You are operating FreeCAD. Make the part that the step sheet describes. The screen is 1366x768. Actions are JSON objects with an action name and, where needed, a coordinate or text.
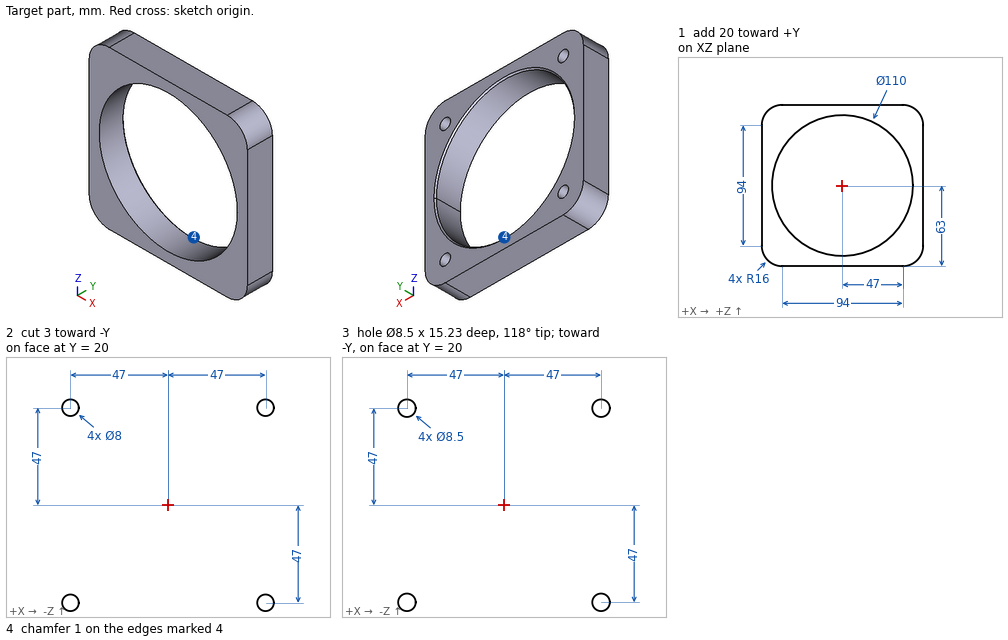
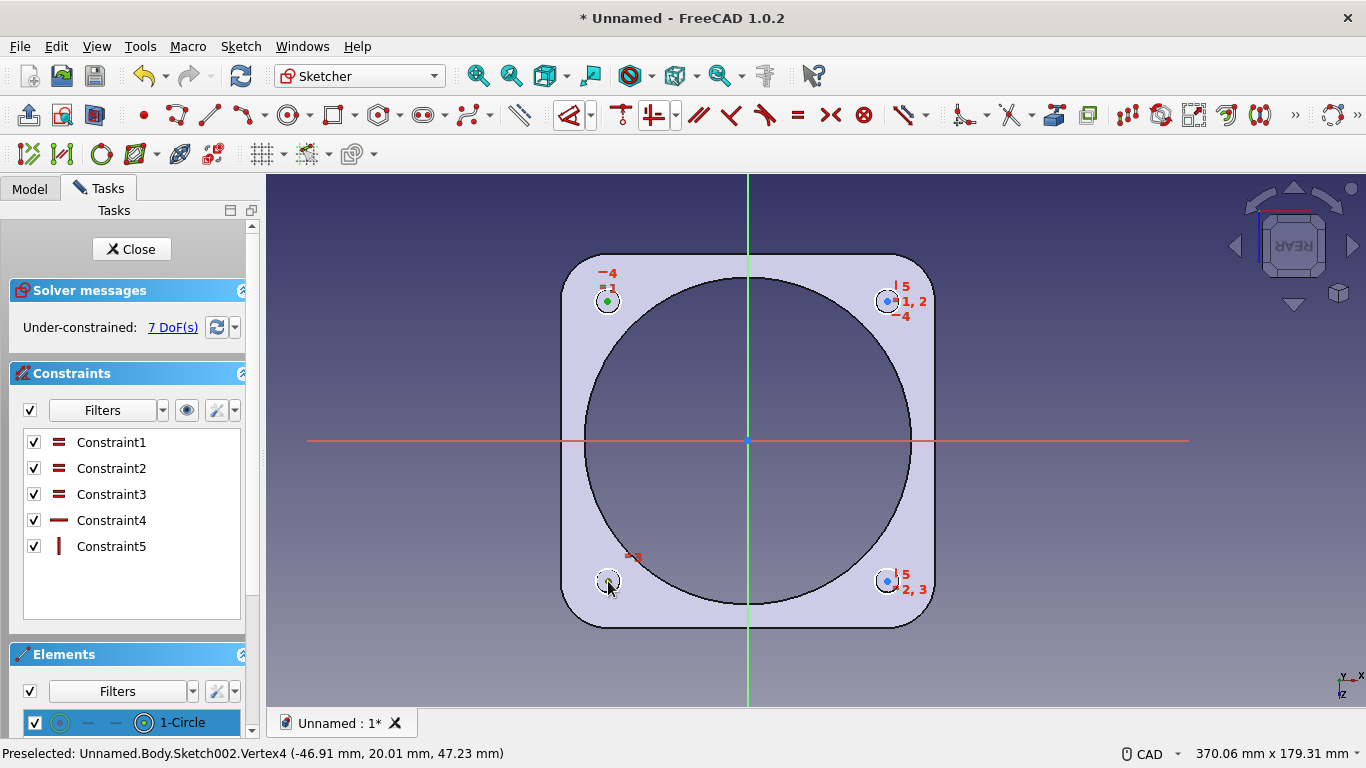
{"action": "key", "text": "v"}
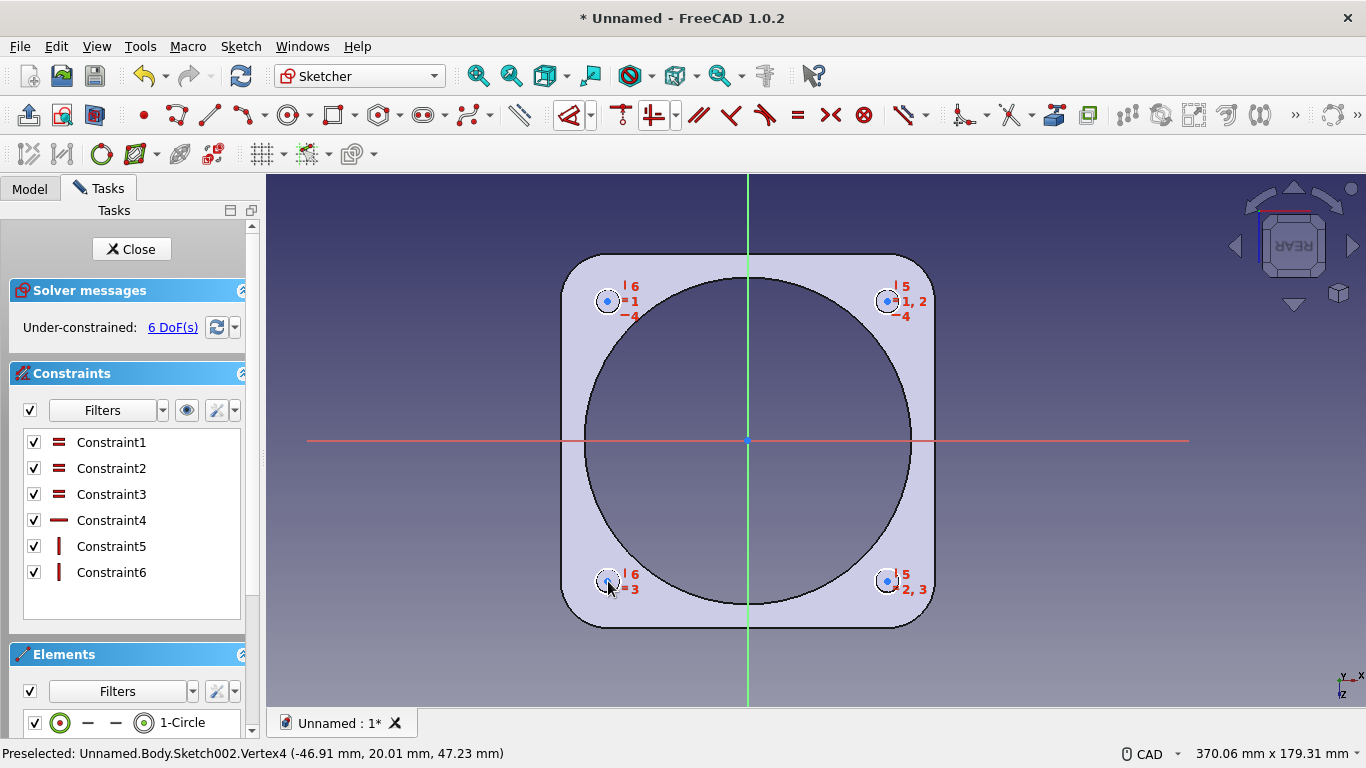
{"action": "left_click", "coordinate": [887, 581]}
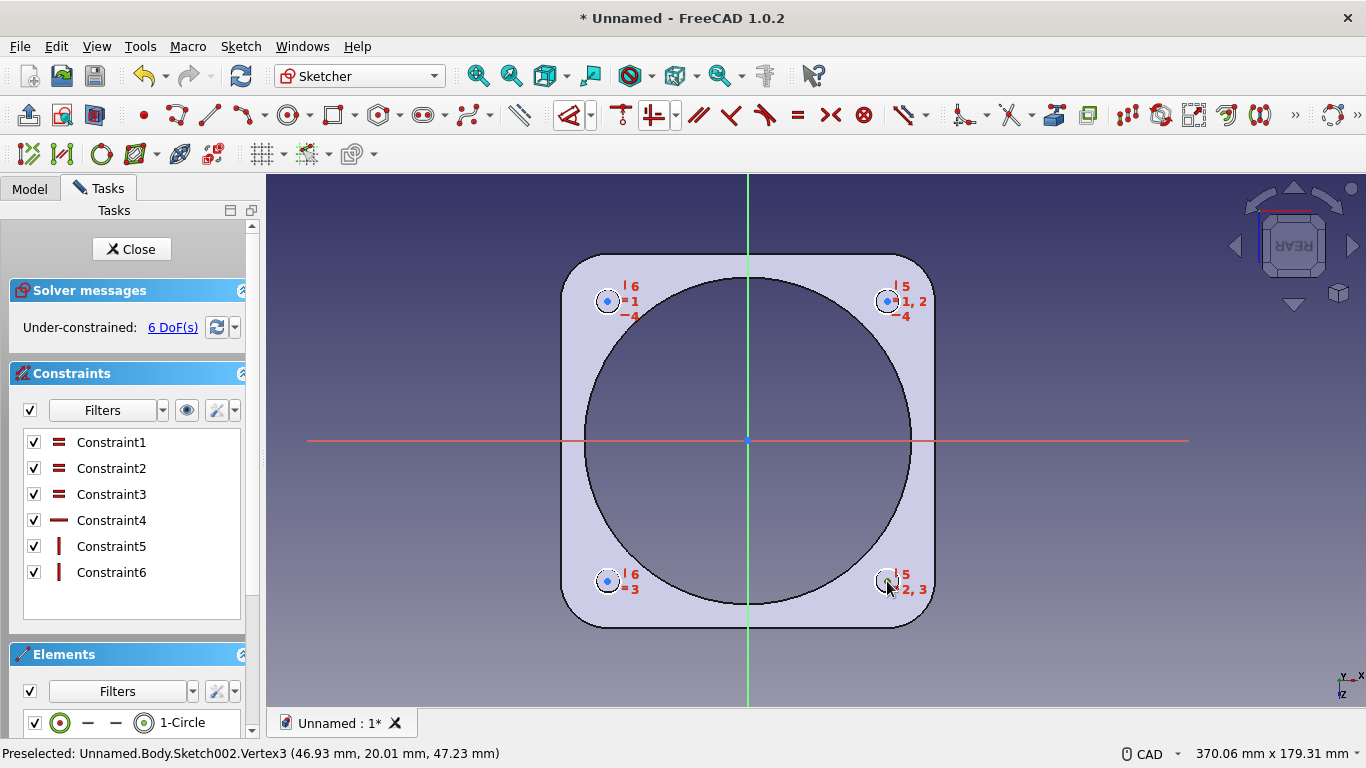
{"action": "left_click", "coordinate": [608, 581]}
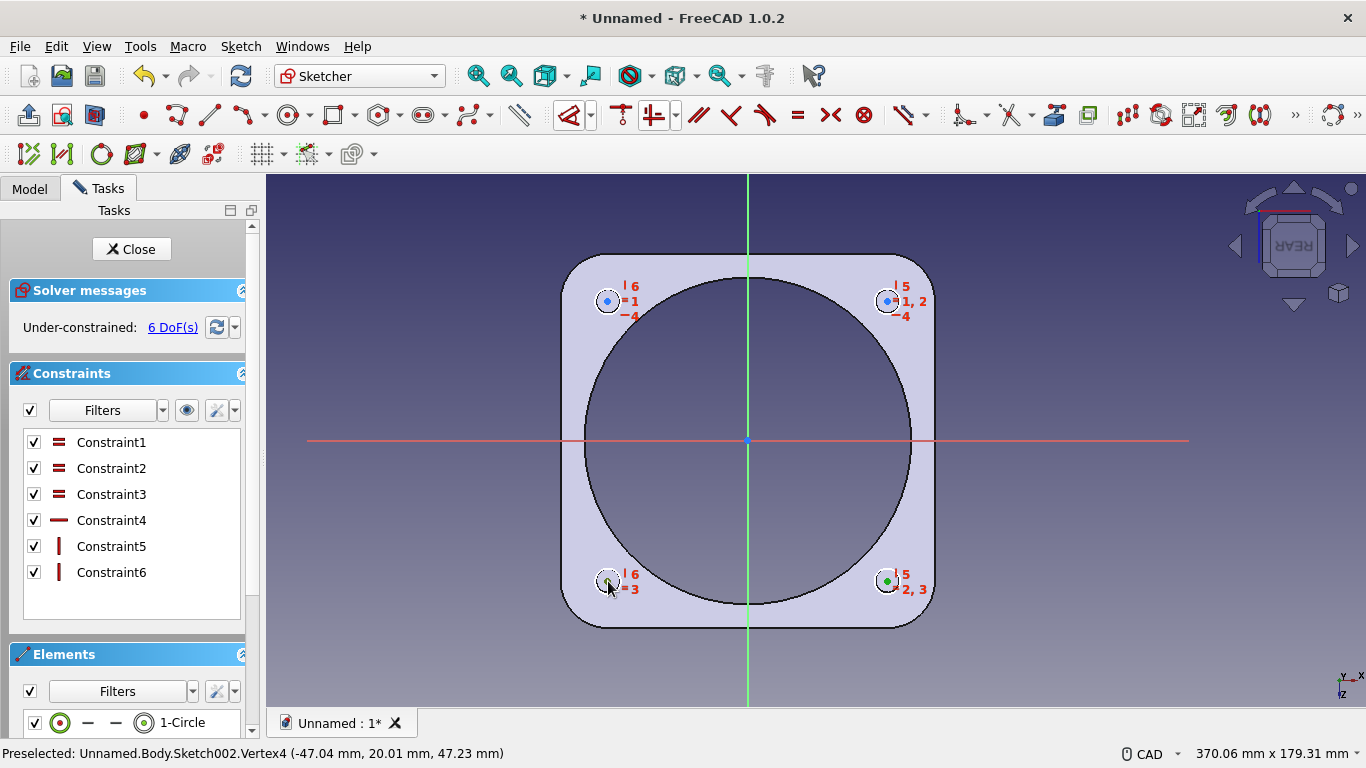
{"action": "key", "text": "h"}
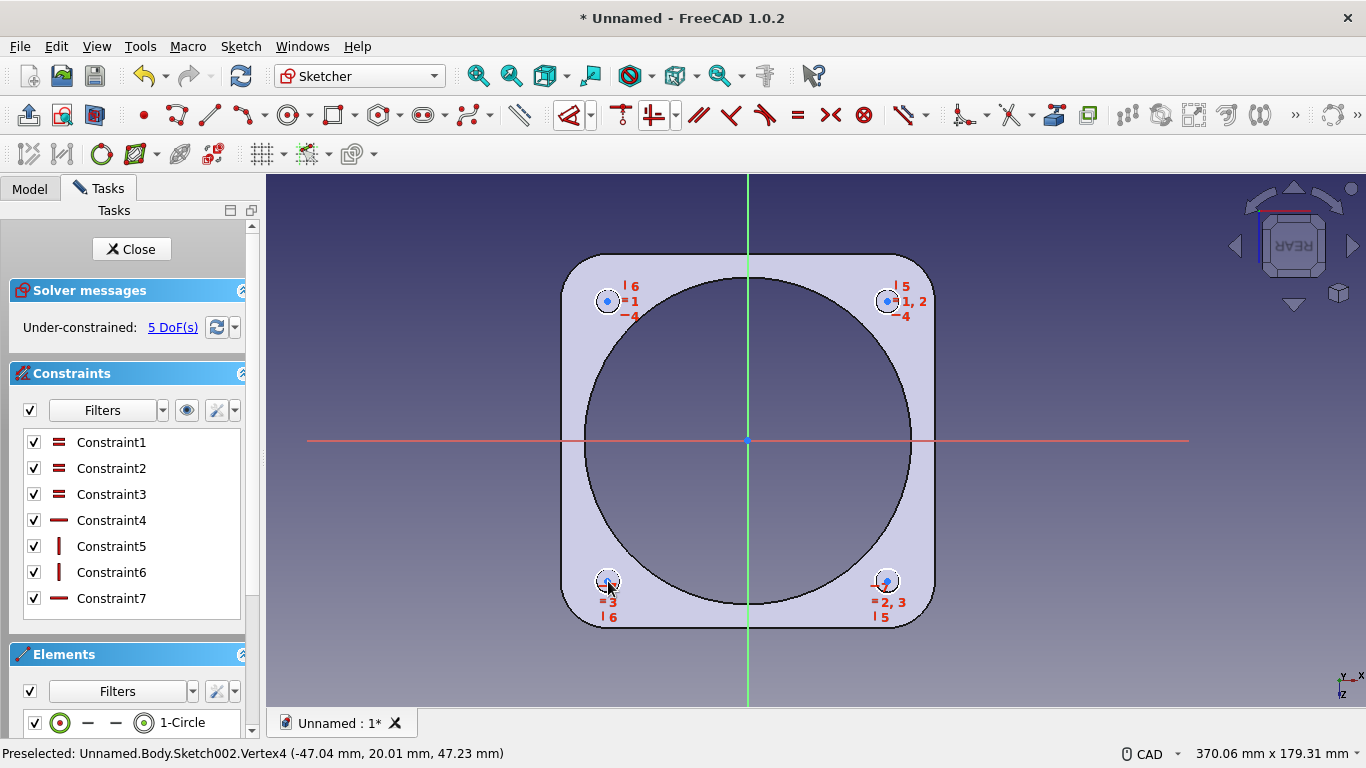
{"action": "scroll", "coordinate": [617, 292], "scroll_direction": "up", "scroll_amount": 3}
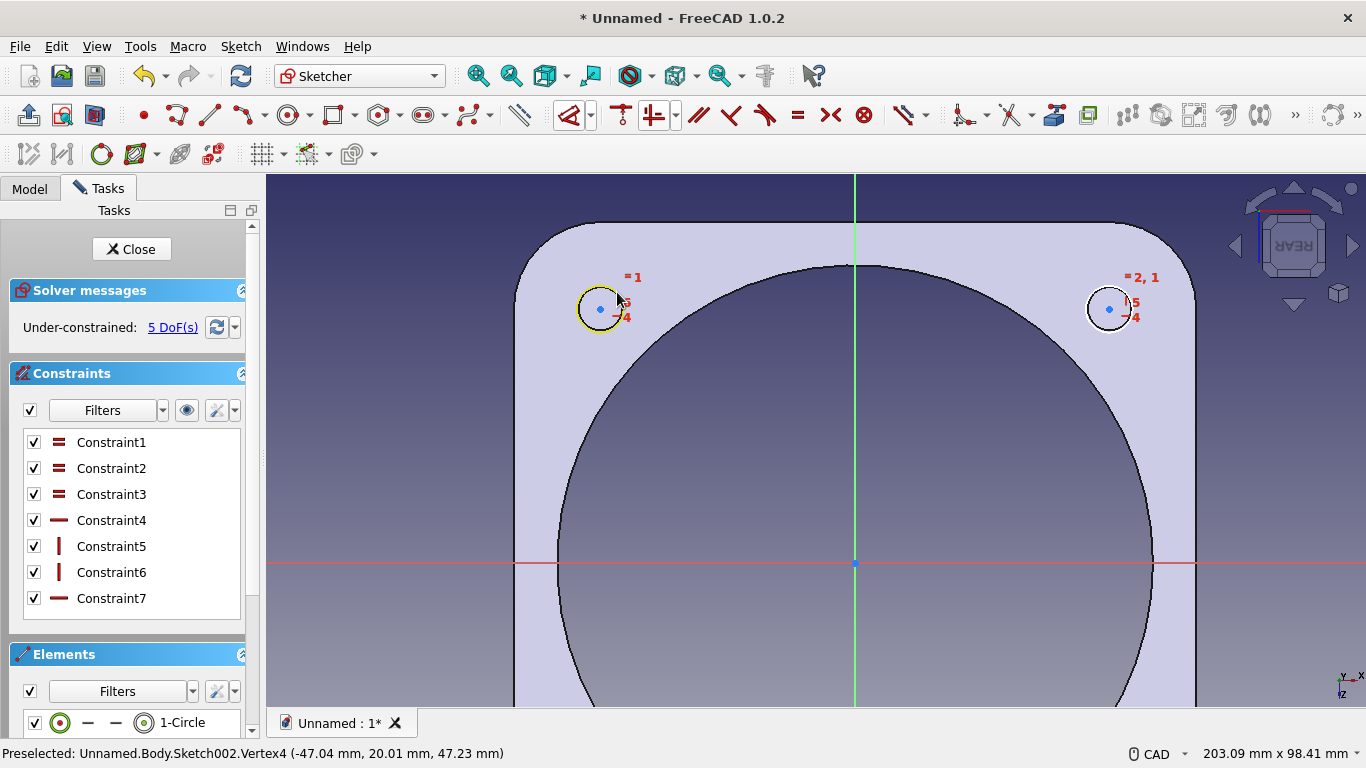
{"action": "left_click", "coordinate": [617, 293]}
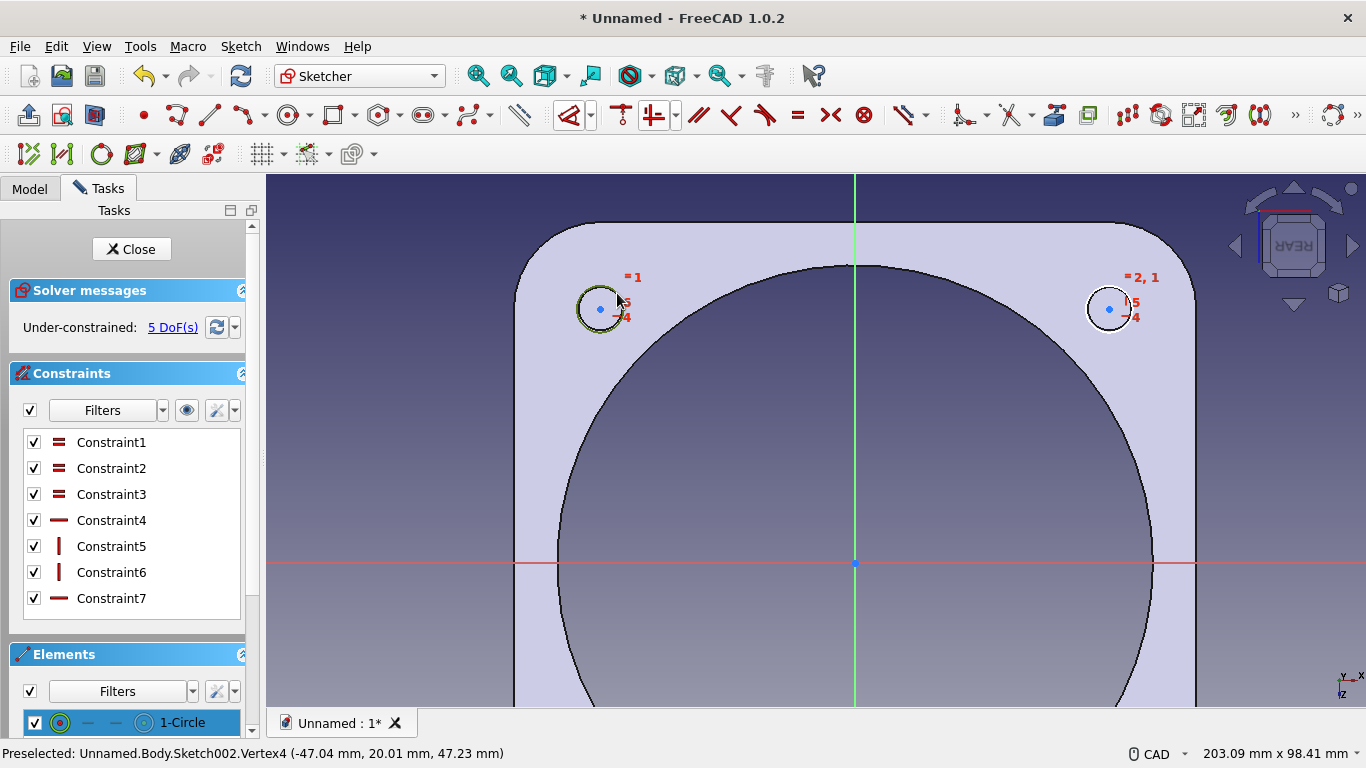
{"action": "key", "text": "k o"}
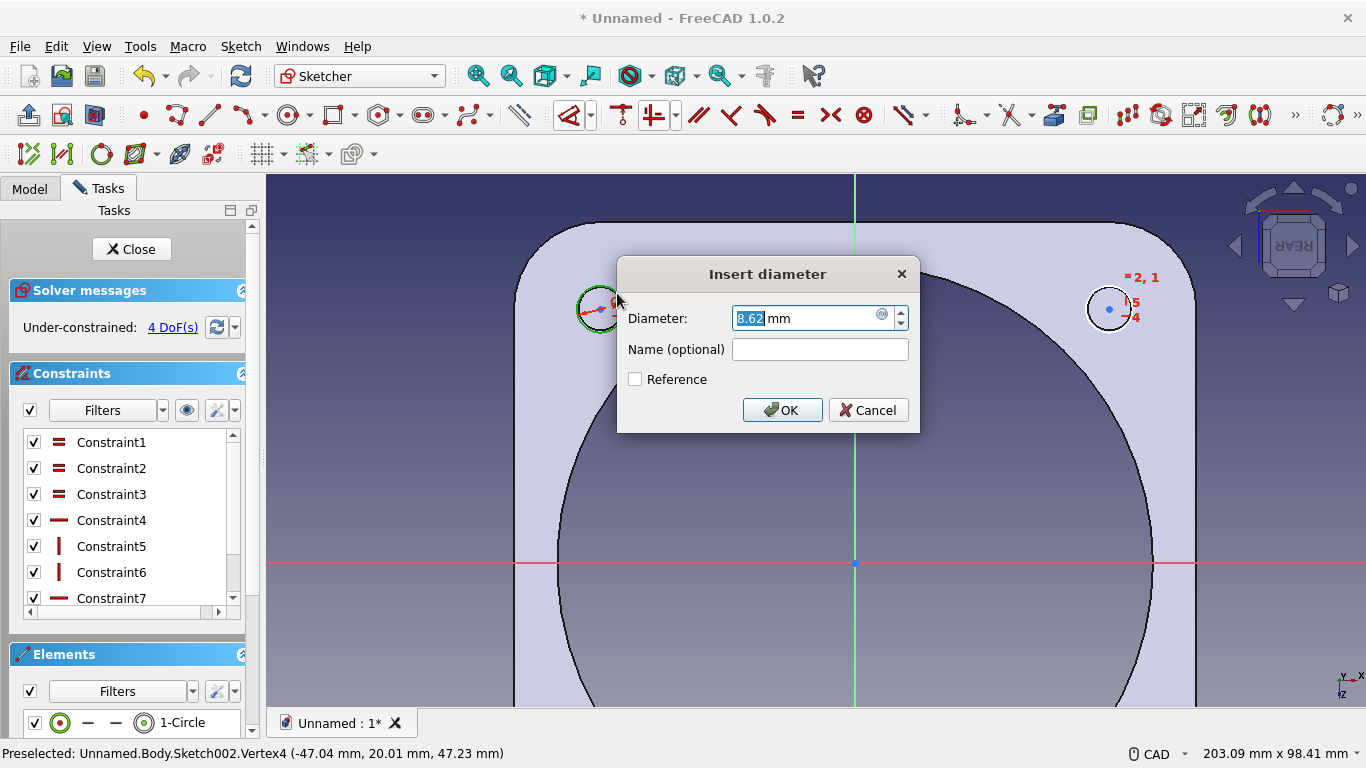
{"action": "type", "text": "8.5"}
{"action": "key", "text": "Return"}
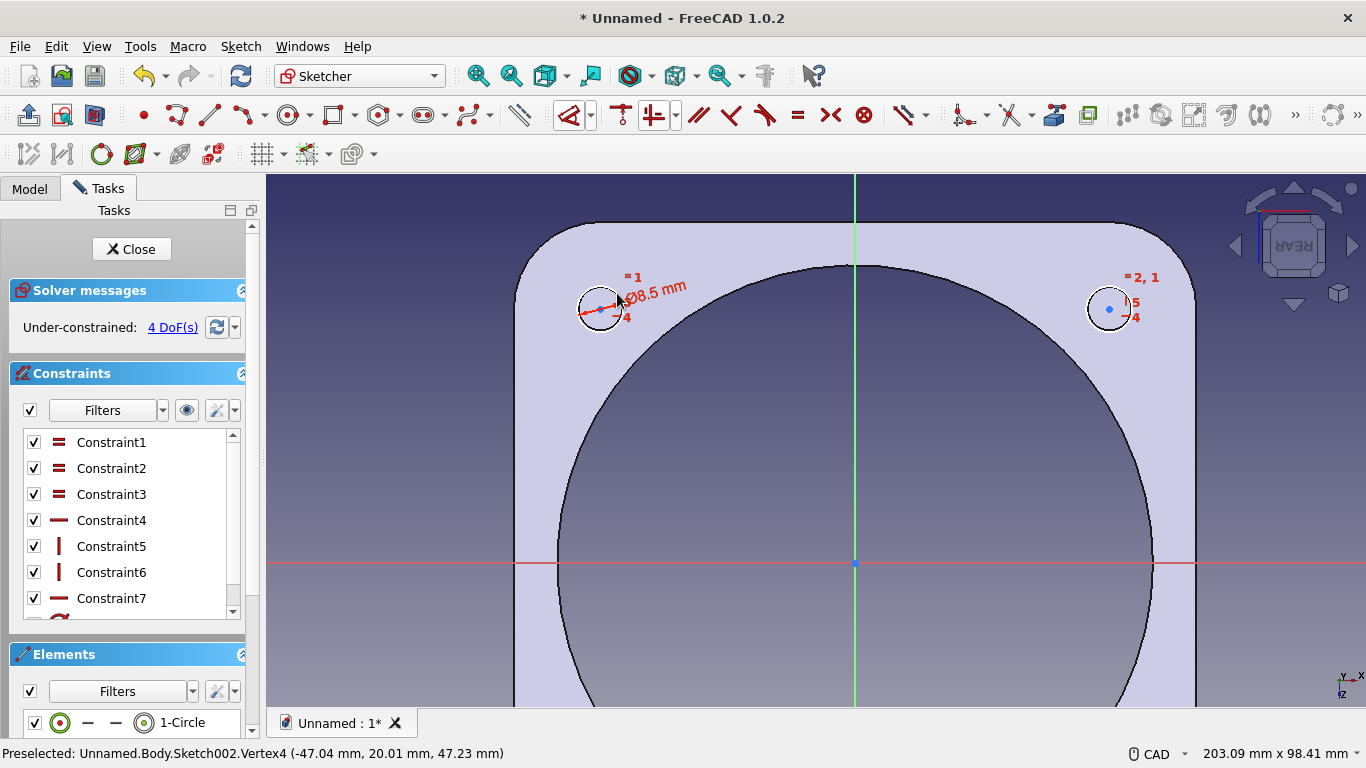
{"action": "left_click", "coordinate": [600, 309]}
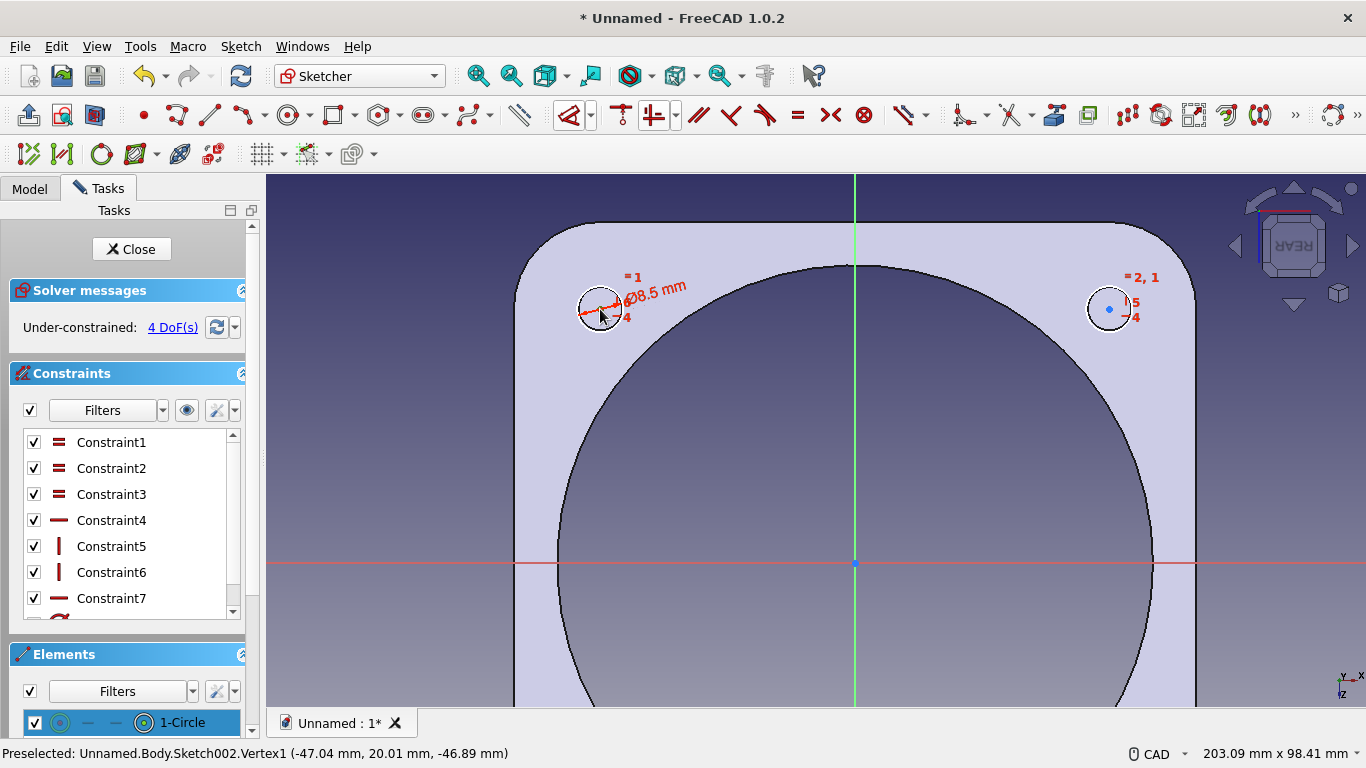
{"action": "left_click", "coordinate": [590, 116]}